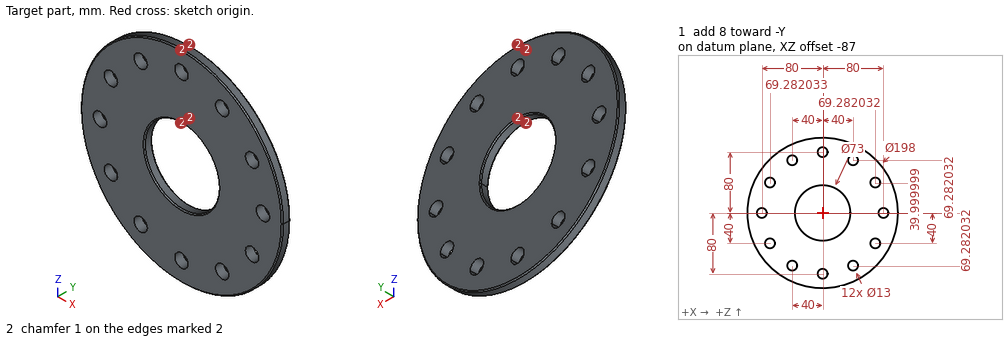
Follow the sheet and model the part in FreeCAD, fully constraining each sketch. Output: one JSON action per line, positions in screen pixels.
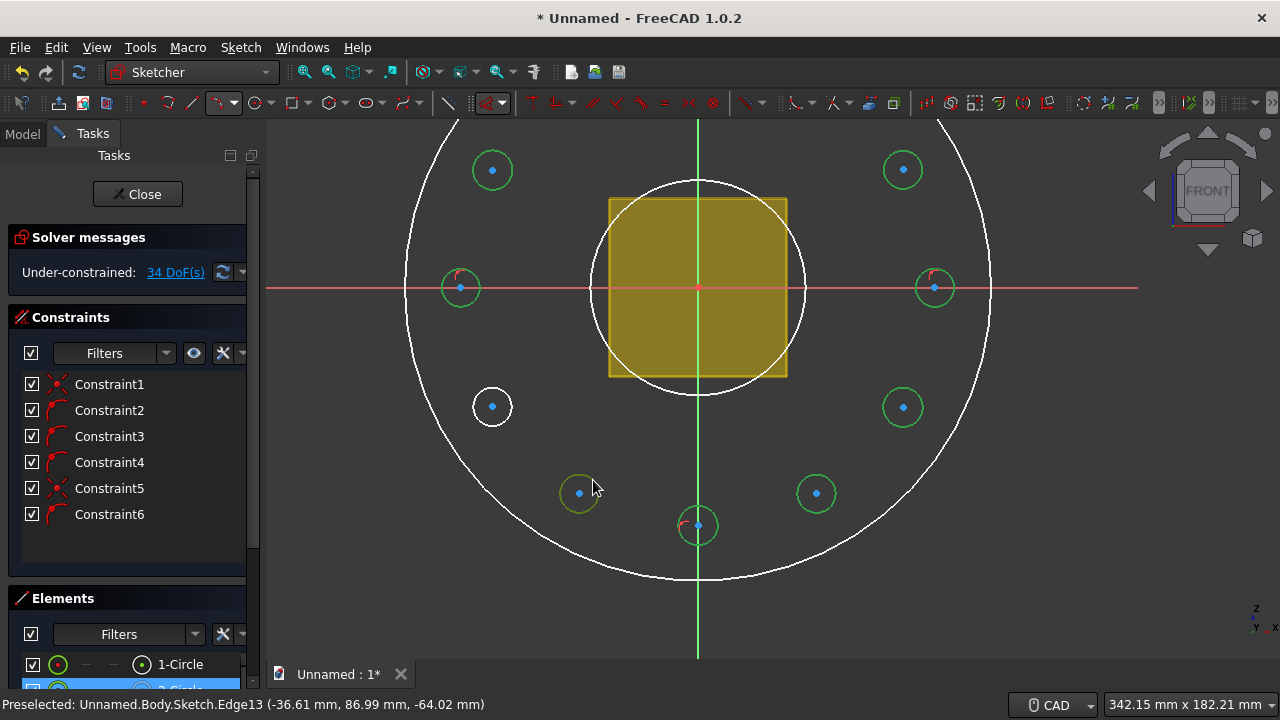
{"action": "left_click", "coordinate": [506, 393]}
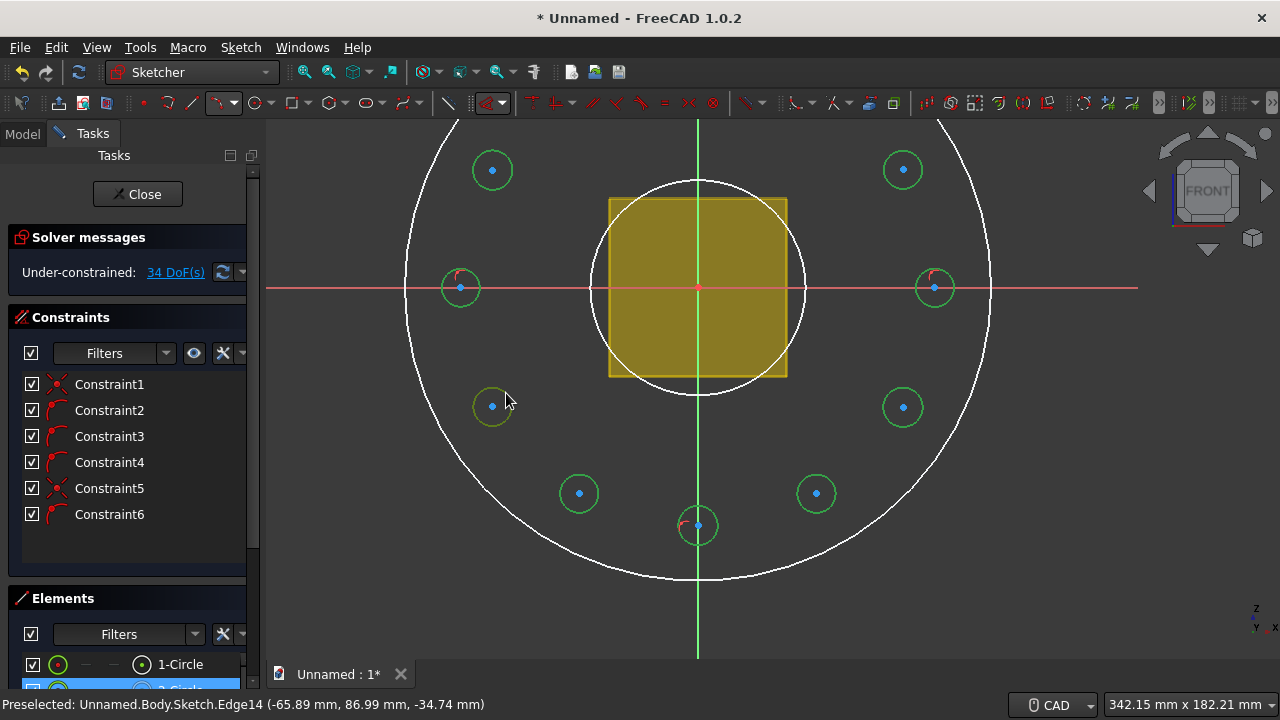
{"action": "key", "text": "e"}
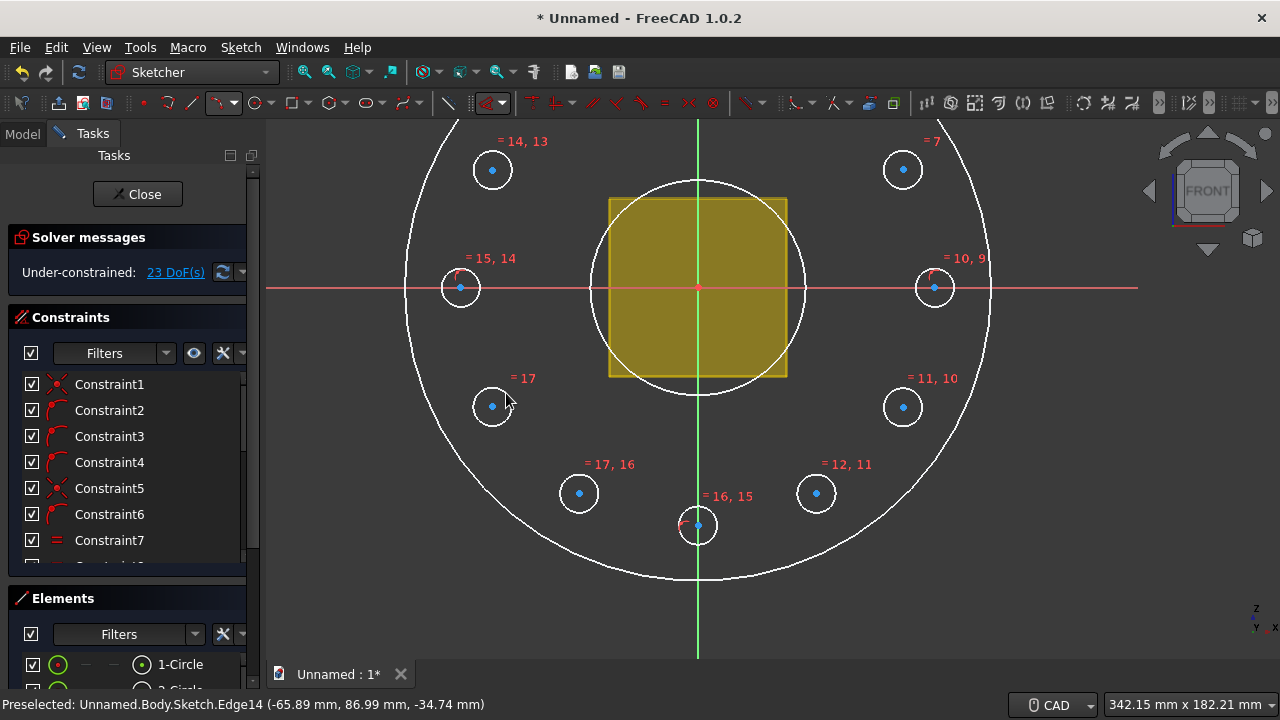
{"action": "left_click", "coordinate": [903, 170]}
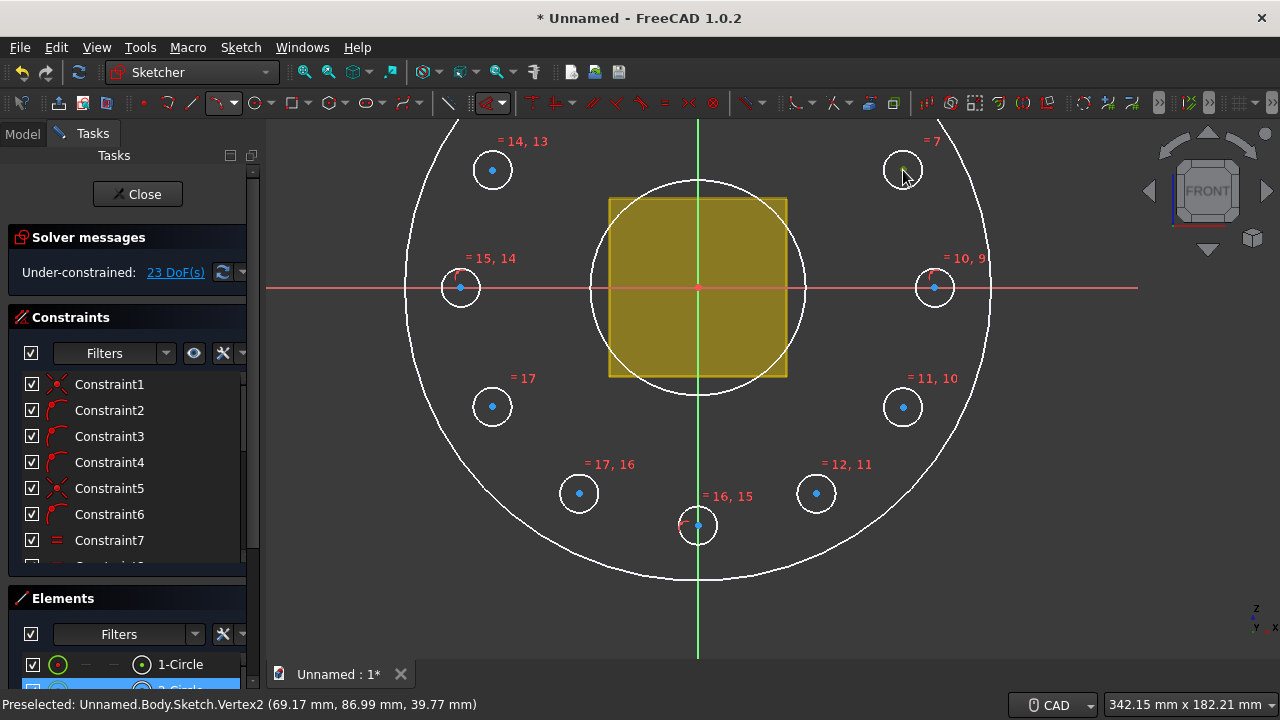
{"action": "left_click", "coordinate": [903, 407]}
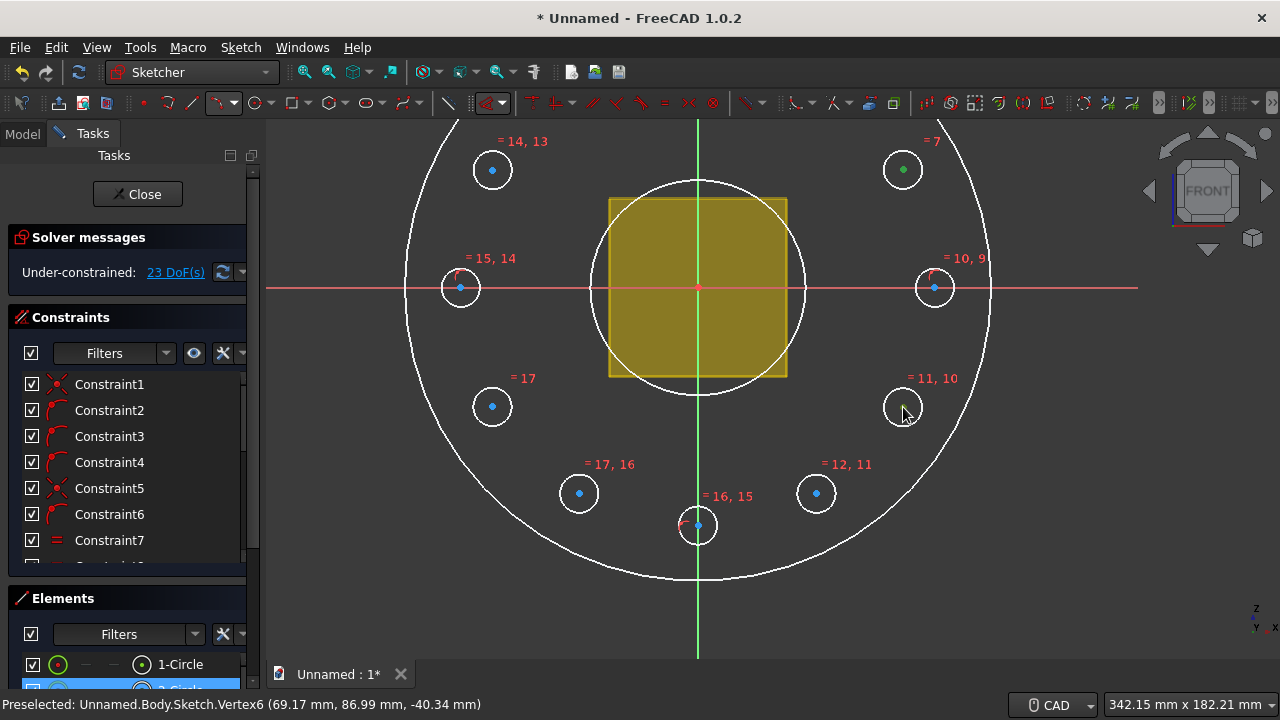
{"action": "key", "text": "v"}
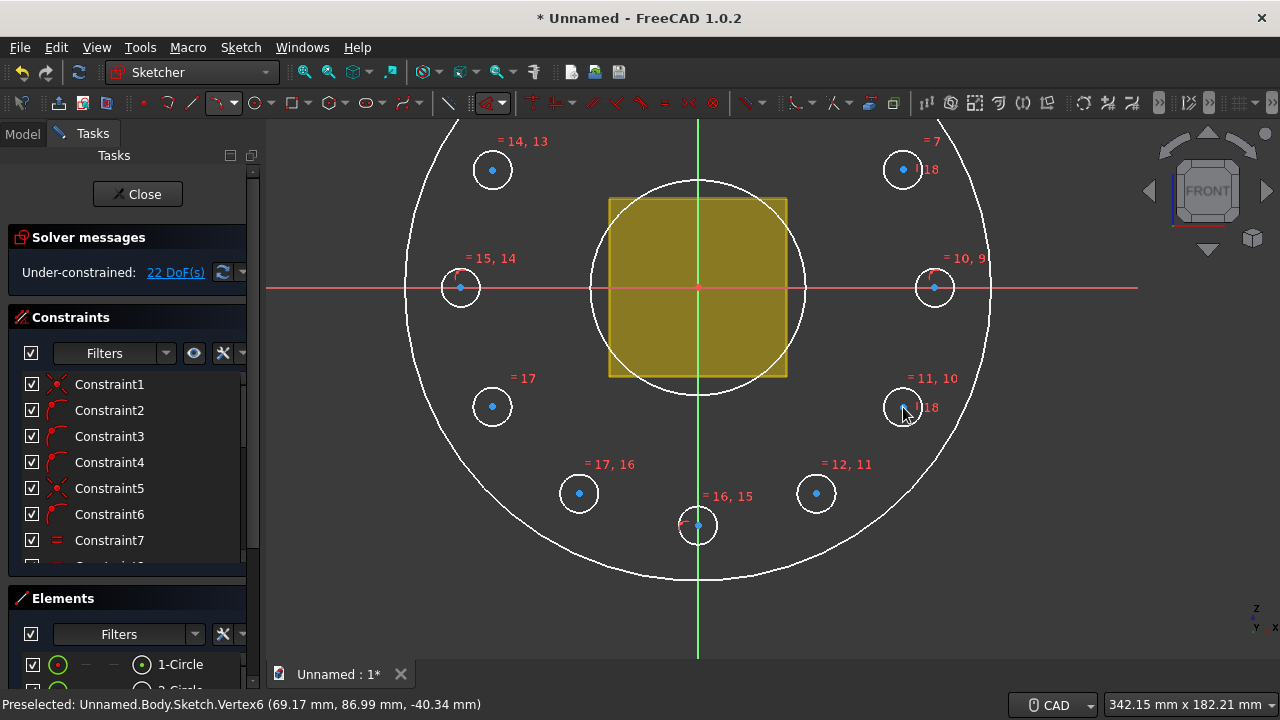
{"action": "scroll", "coordinate": [712, 512], "scroll_direction": "down", "scroll_amount": 3}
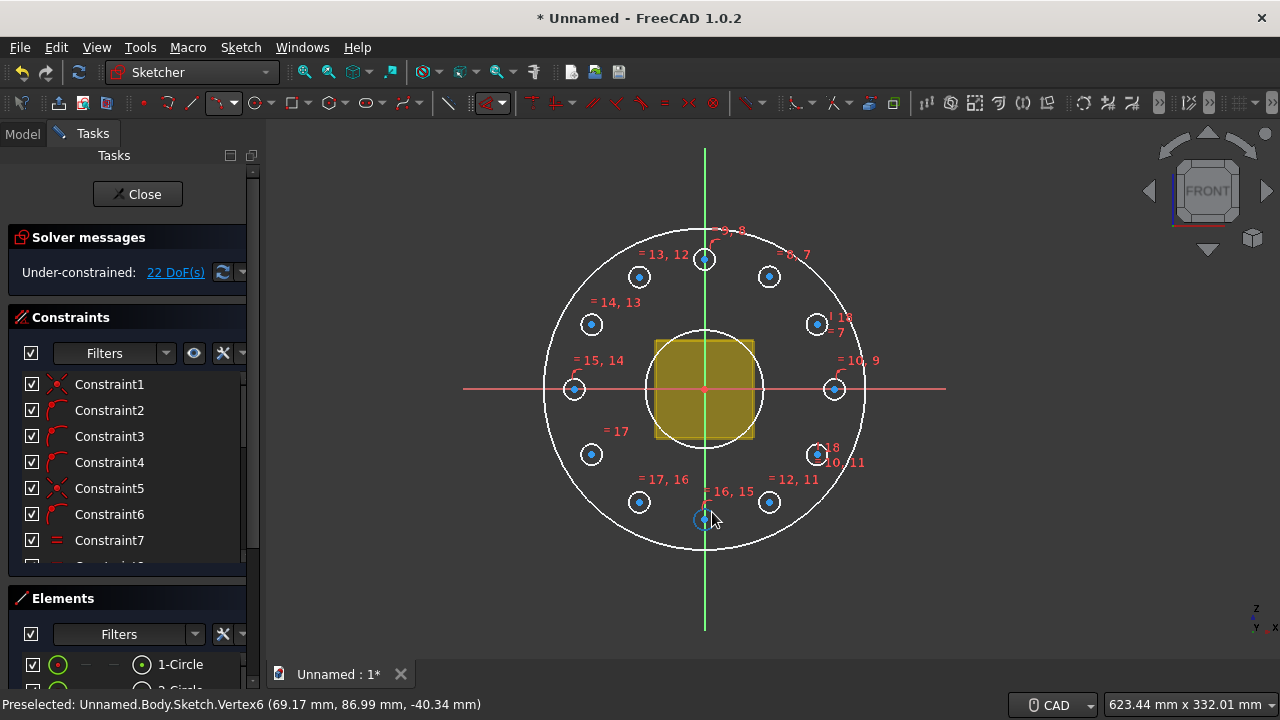
{"action": "left_click", "coordinate": [769, 277]}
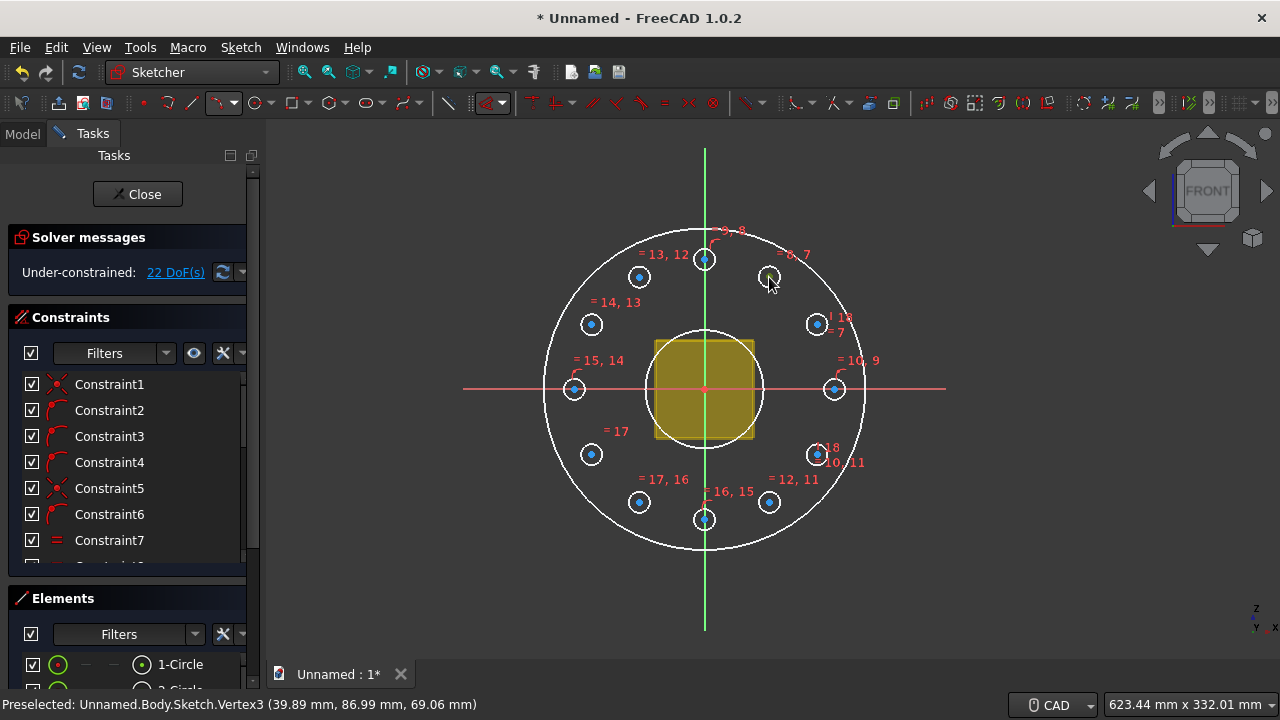
{"action": "left_click", "coordinate": [770, 502]}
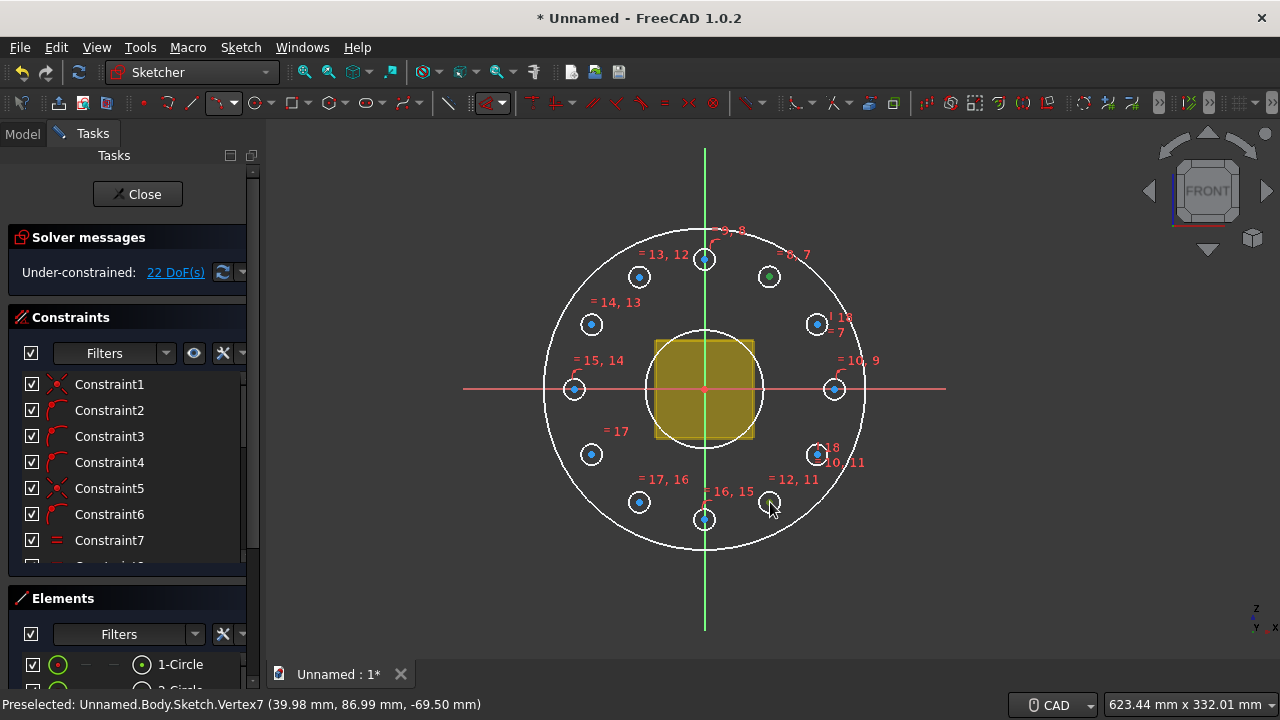
{"action": "key", "text": "v"}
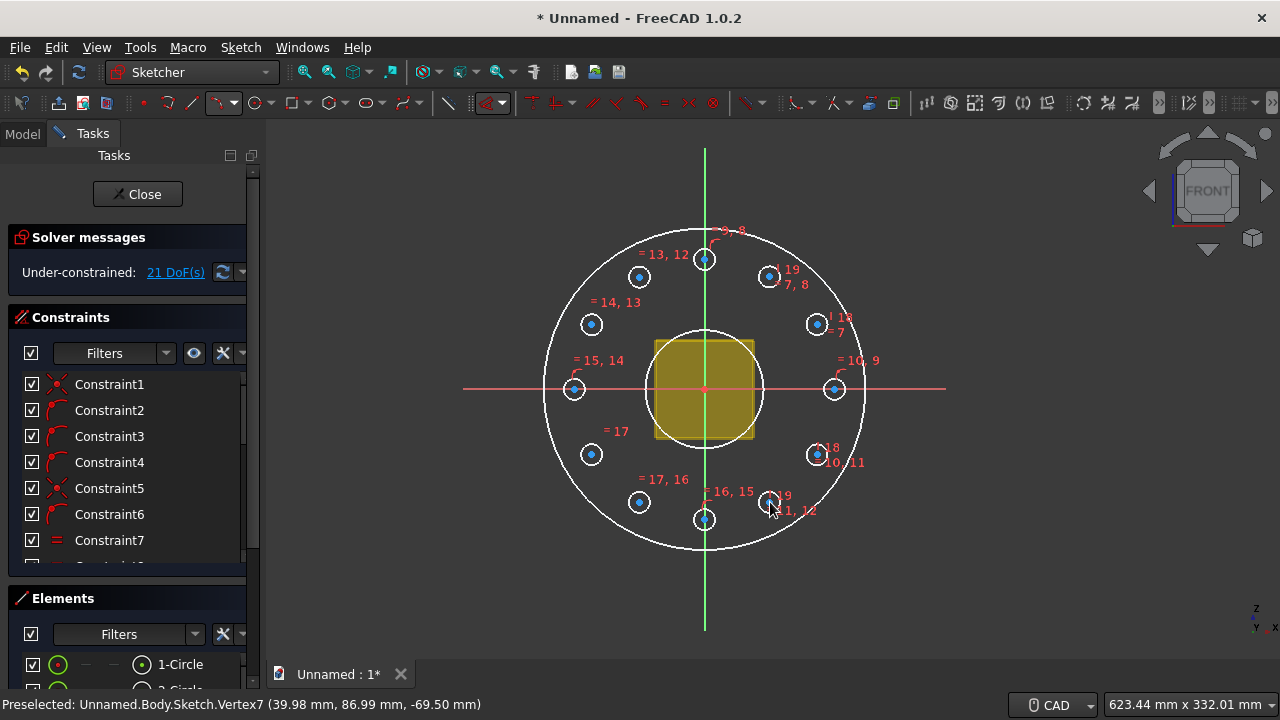
{"action": "left_click", "coordinate": [769, 277]}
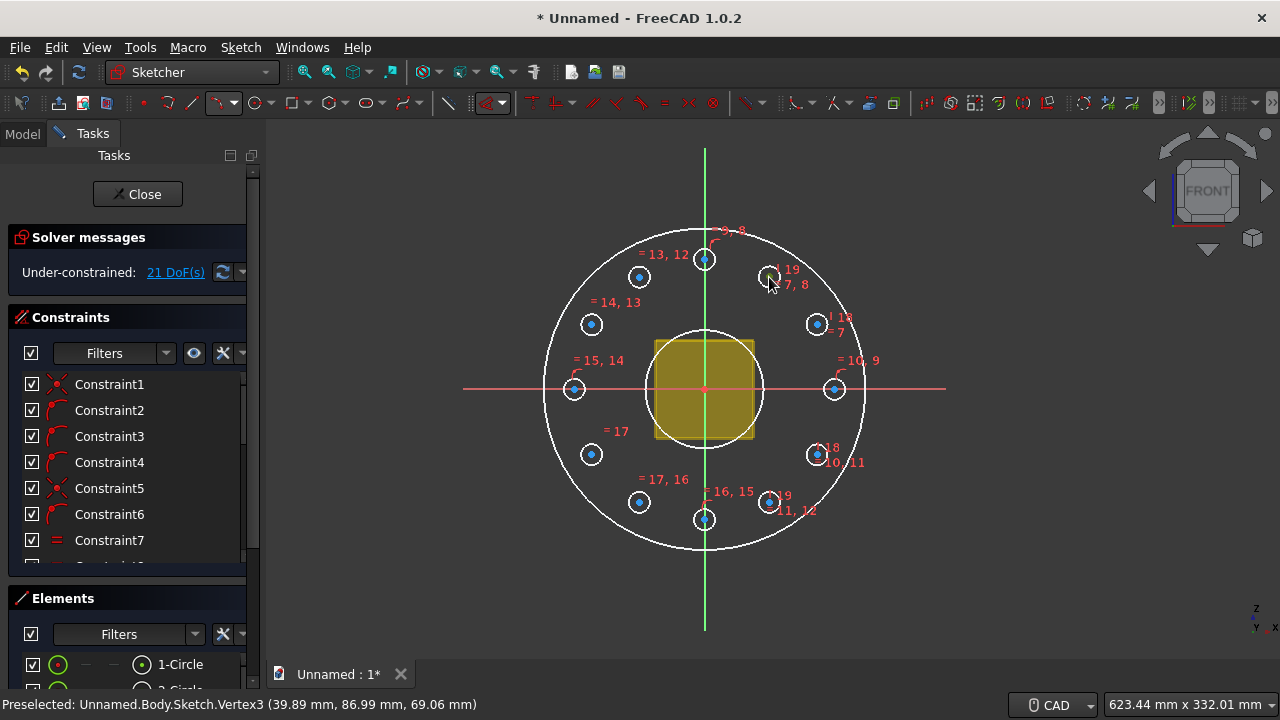
{"action": "left_click", "coordinate": [639, 277]}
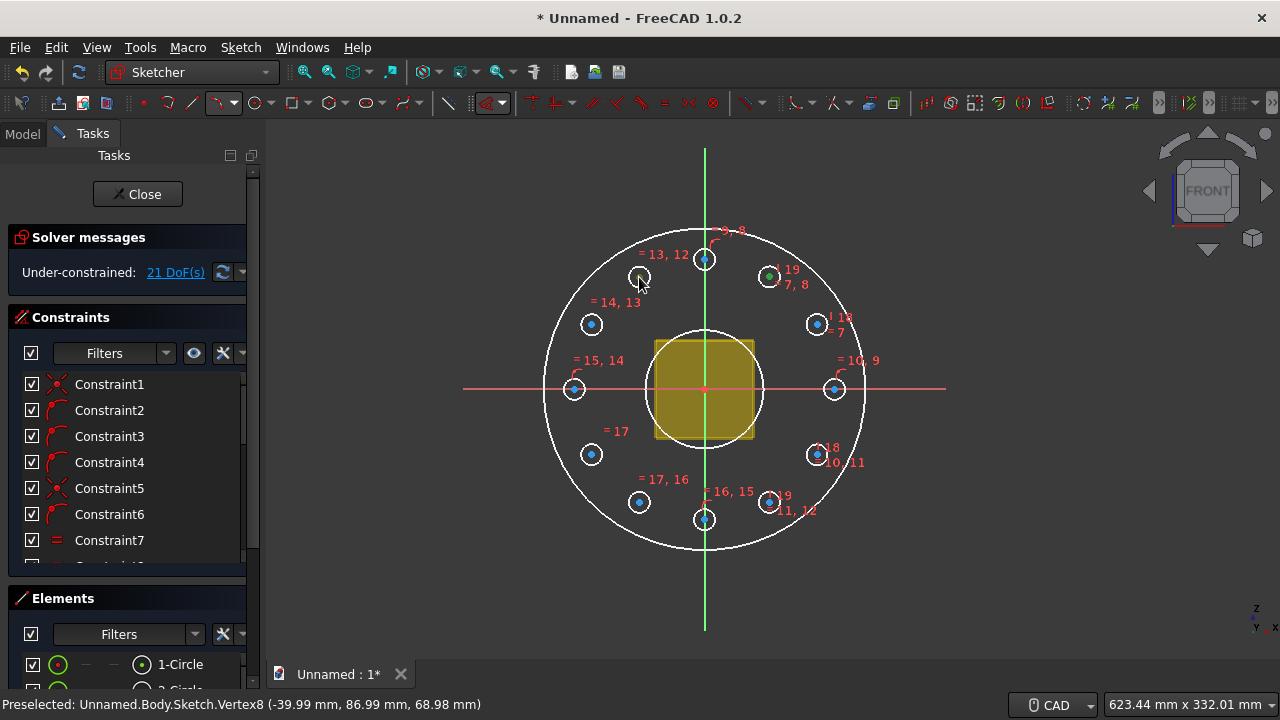
{"action": "key", "text": "h"}